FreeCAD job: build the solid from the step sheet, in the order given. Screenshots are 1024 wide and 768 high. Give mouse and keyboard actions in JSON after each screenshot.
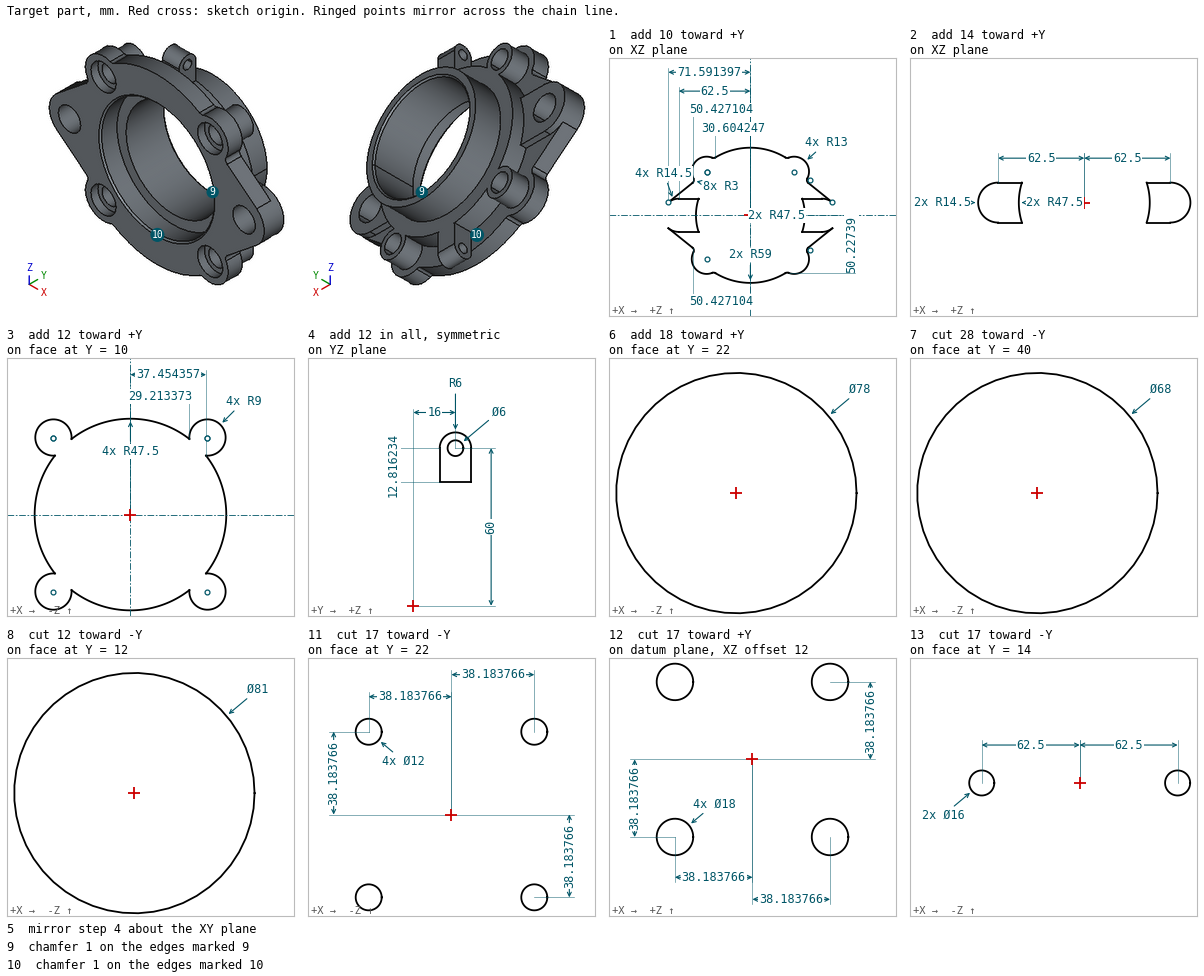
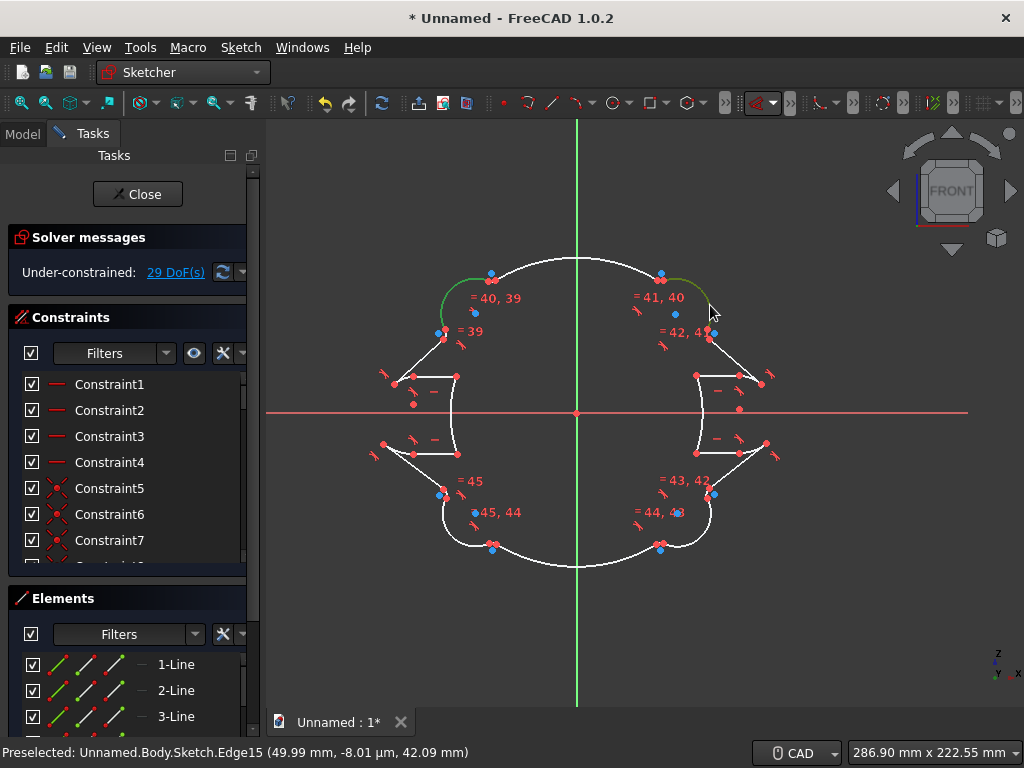
{"action": "left_click", "coordinate": [688, 545]}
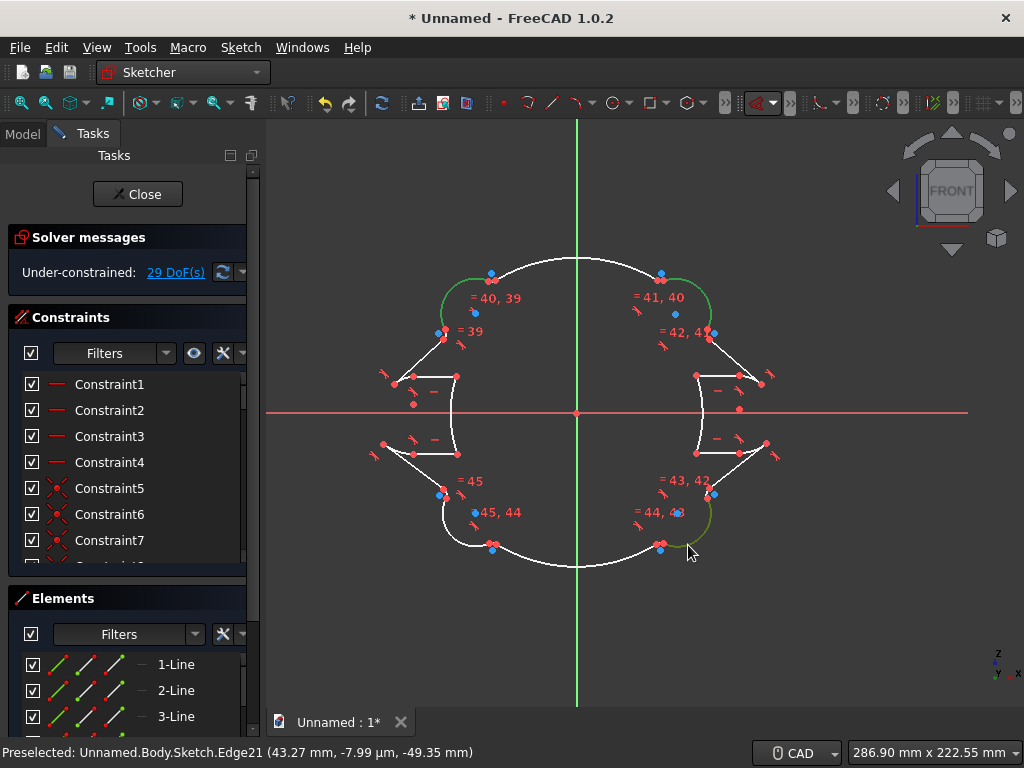
{"action": "left_click", "coordinate": [444, 522]}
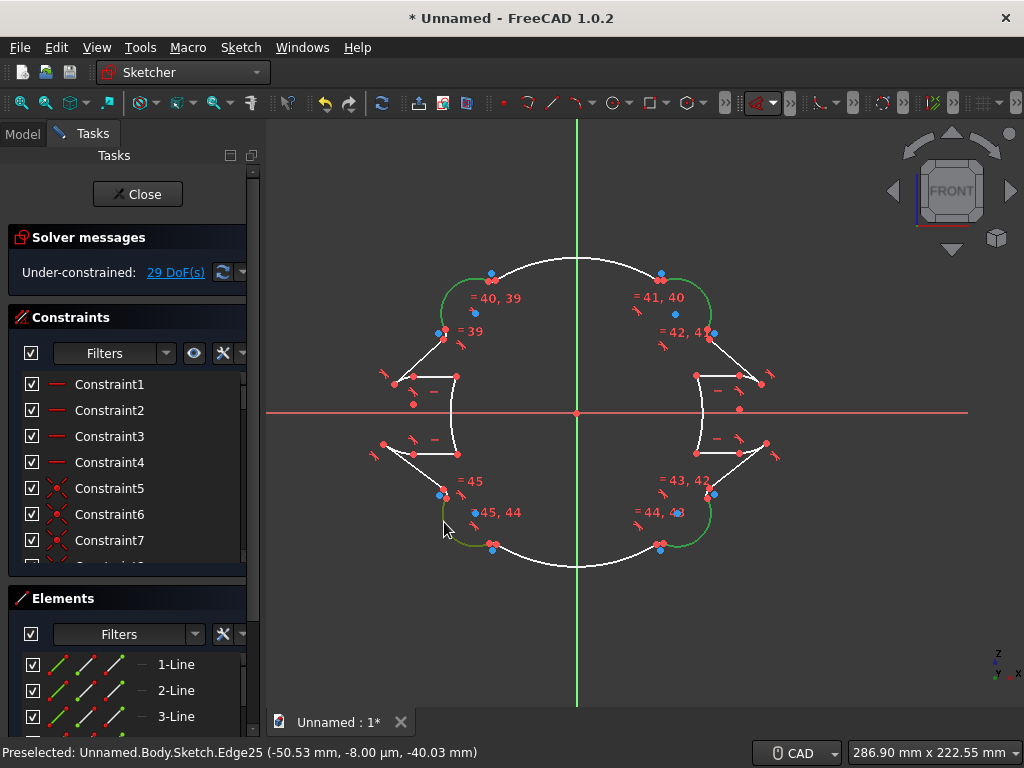
{"action": "key", "text": "e"}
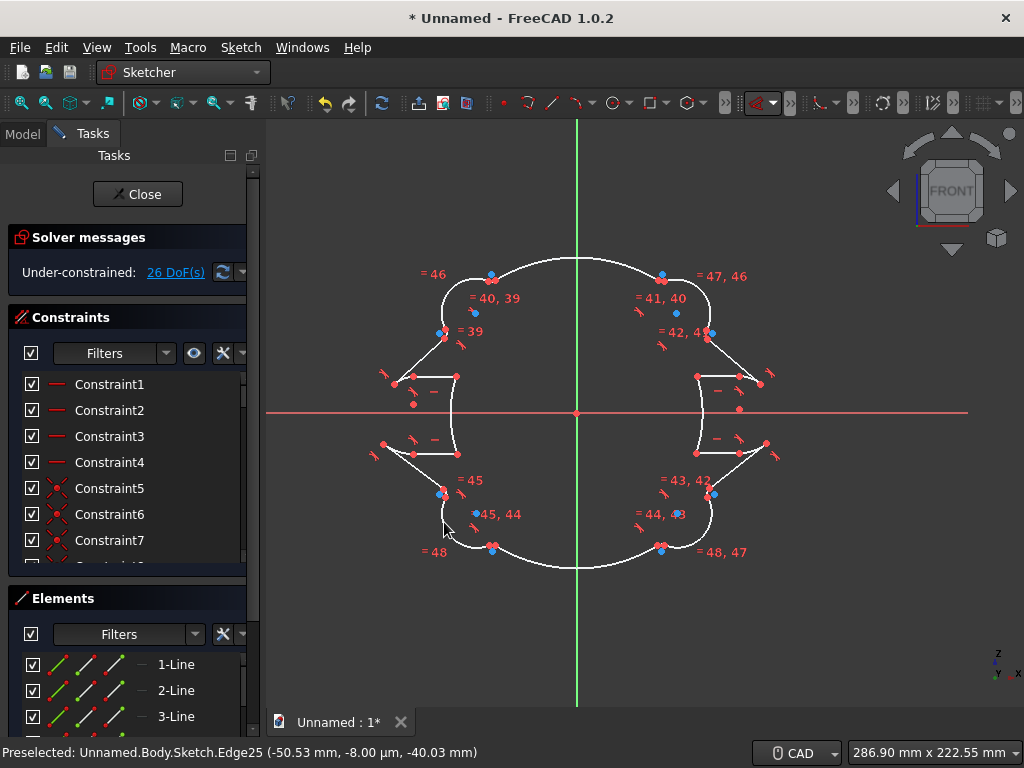
{"action": "scroll", "coordinate": [409, 377], "scroll_direction": "up", "scroll_amount": 7}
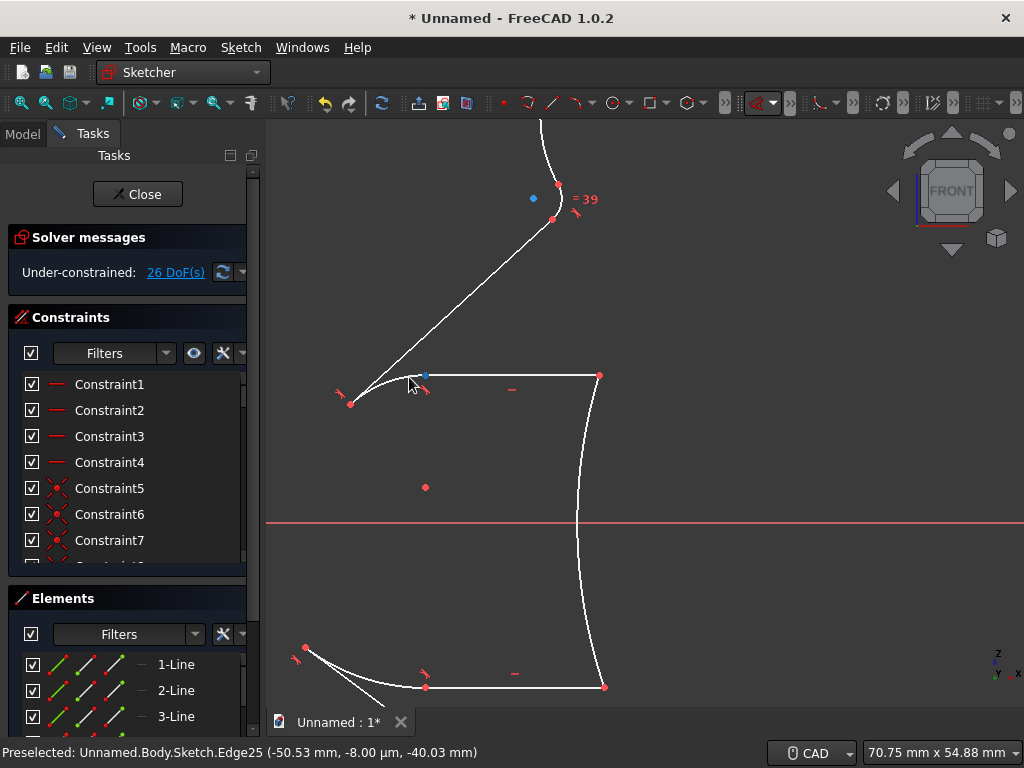
{"action": "left_click", "coordinate": [409, 376]}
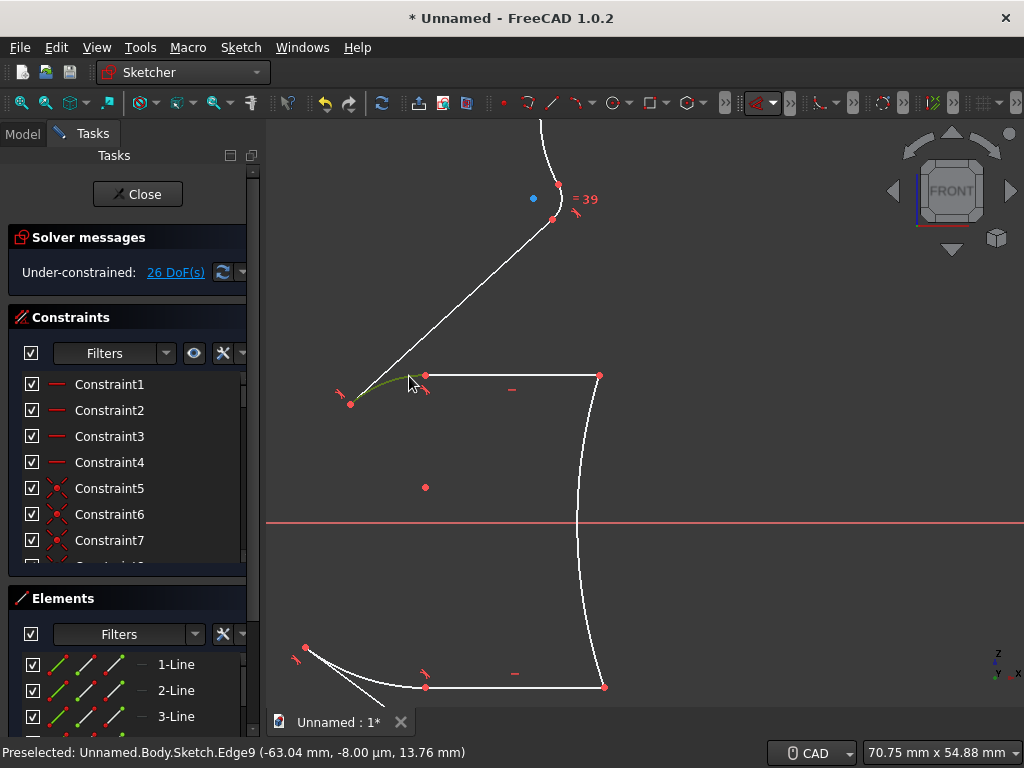
{"action": "scroll", "coordinate": [409, 377], "scroll_direction": "down", "scroll_amount": 7}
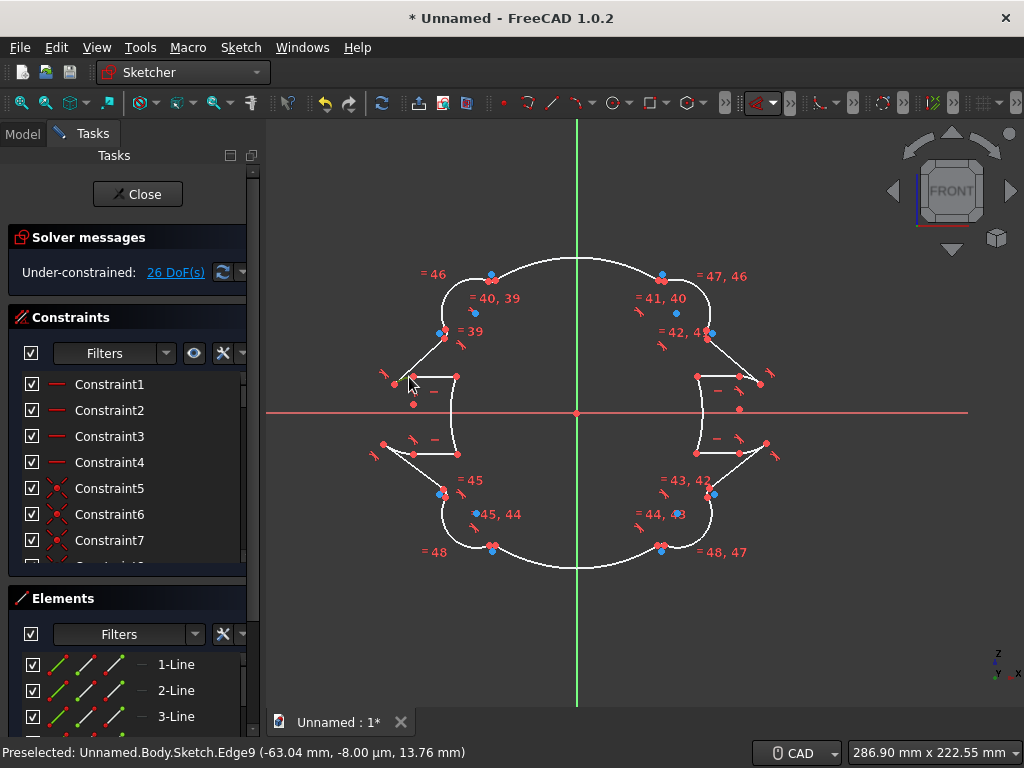
{"action": "scroll", "coordinate": [746, 377], "scroll_direction": "up", "scroll_amount": 7}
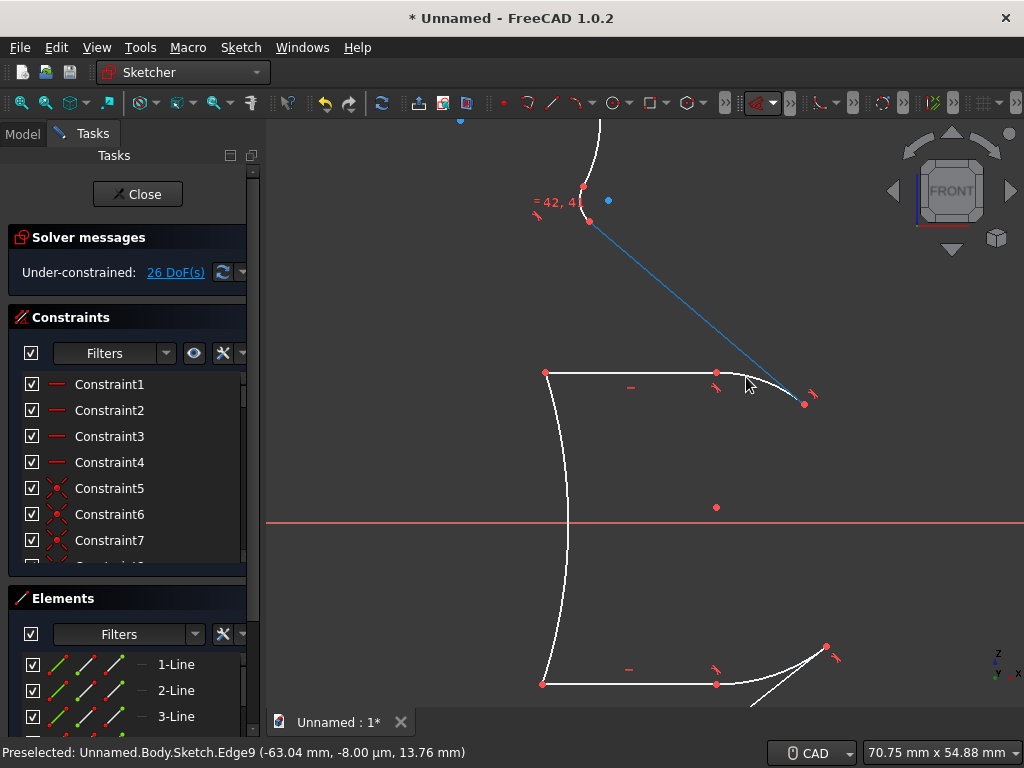
{"action": "left_click", "coordinate": [745, 376]}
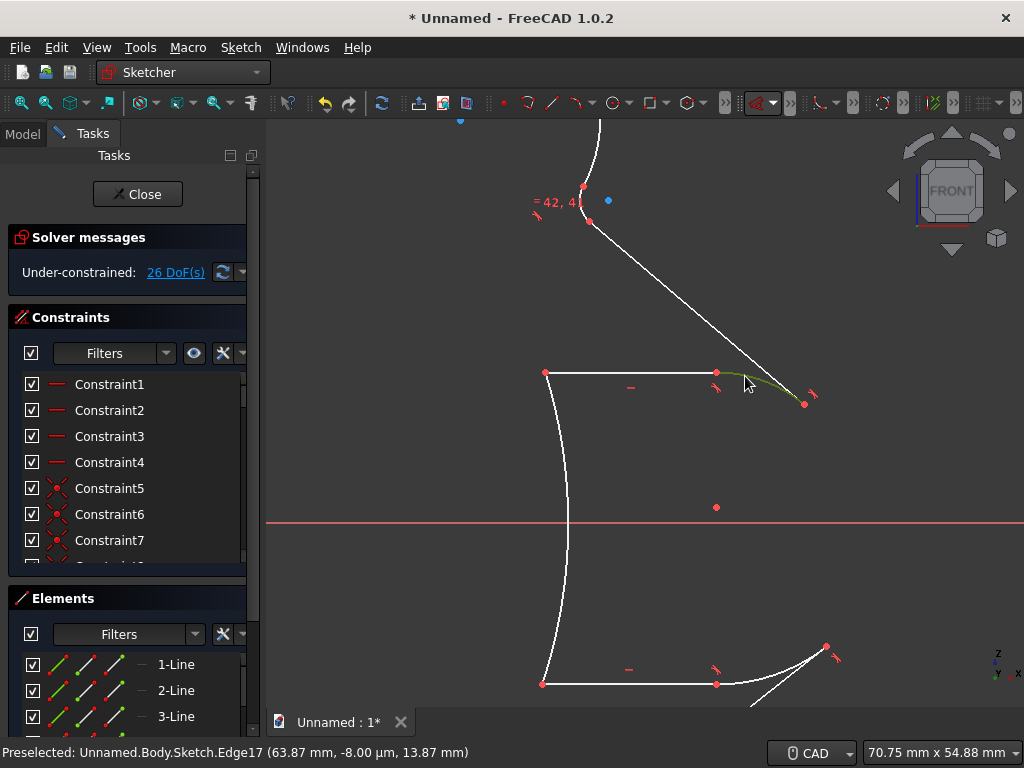
{"action": "scroll", "coordinate": [775, 675], "scroll_direction": "up", "scroll_amount": 2}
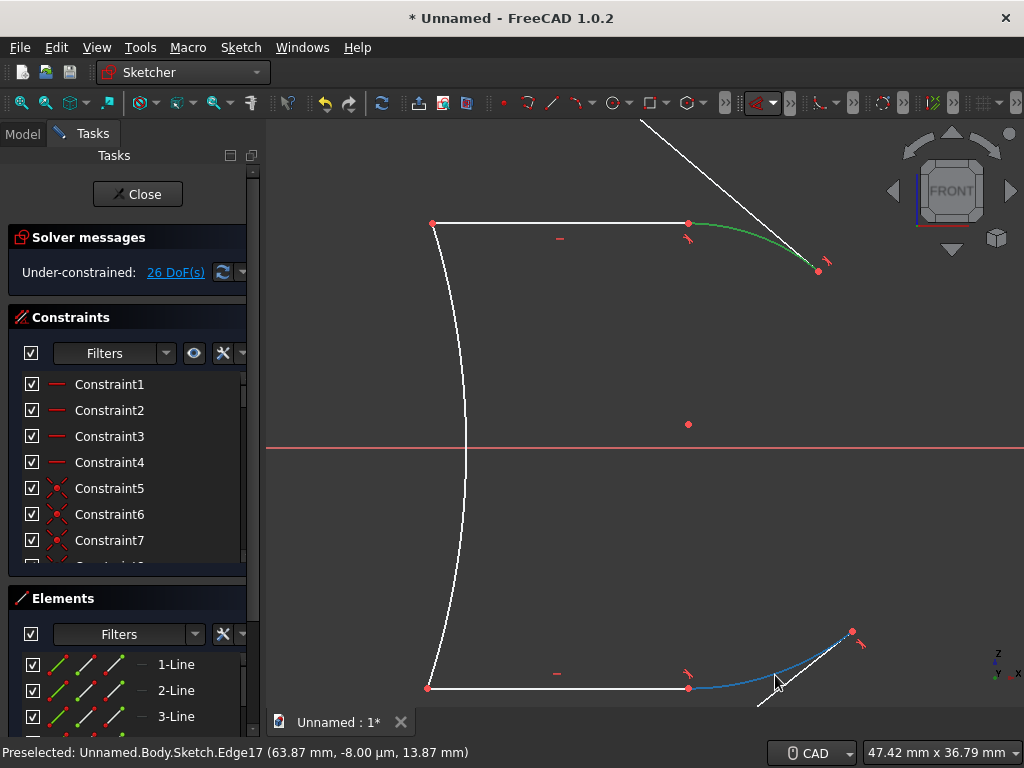
{"action": "left_click", "coordinate": [775, 674]}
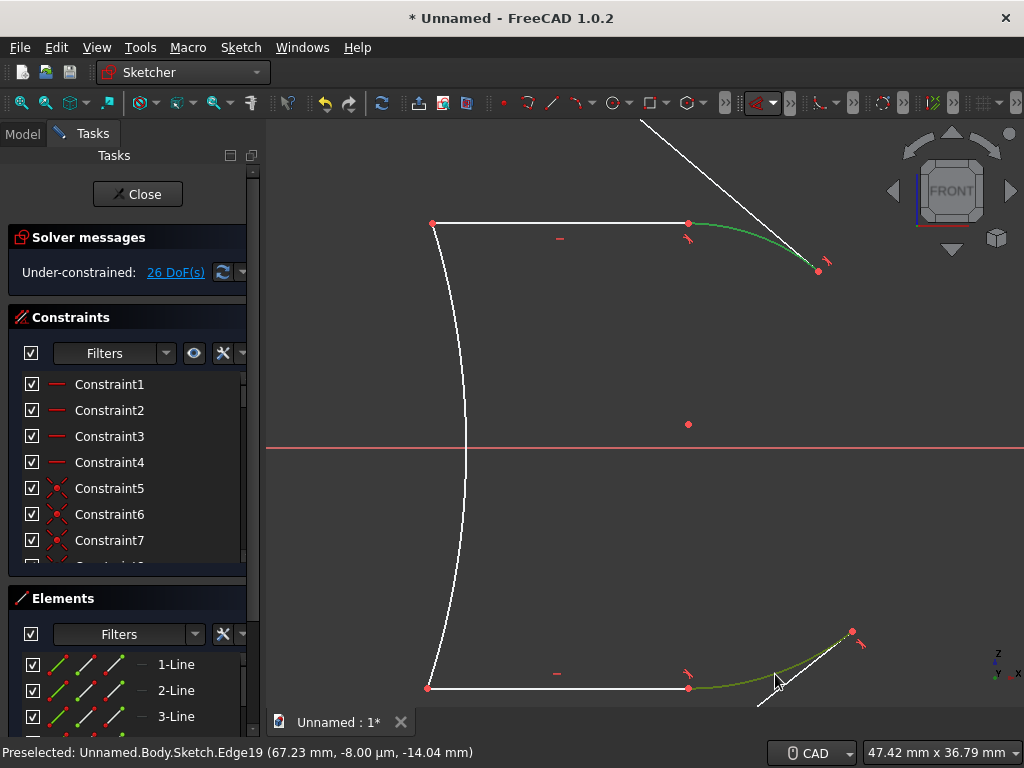
{"action": "scroll", "coordinate": [749, 406], "scroll_direction": "down", "scroll_amount": 9}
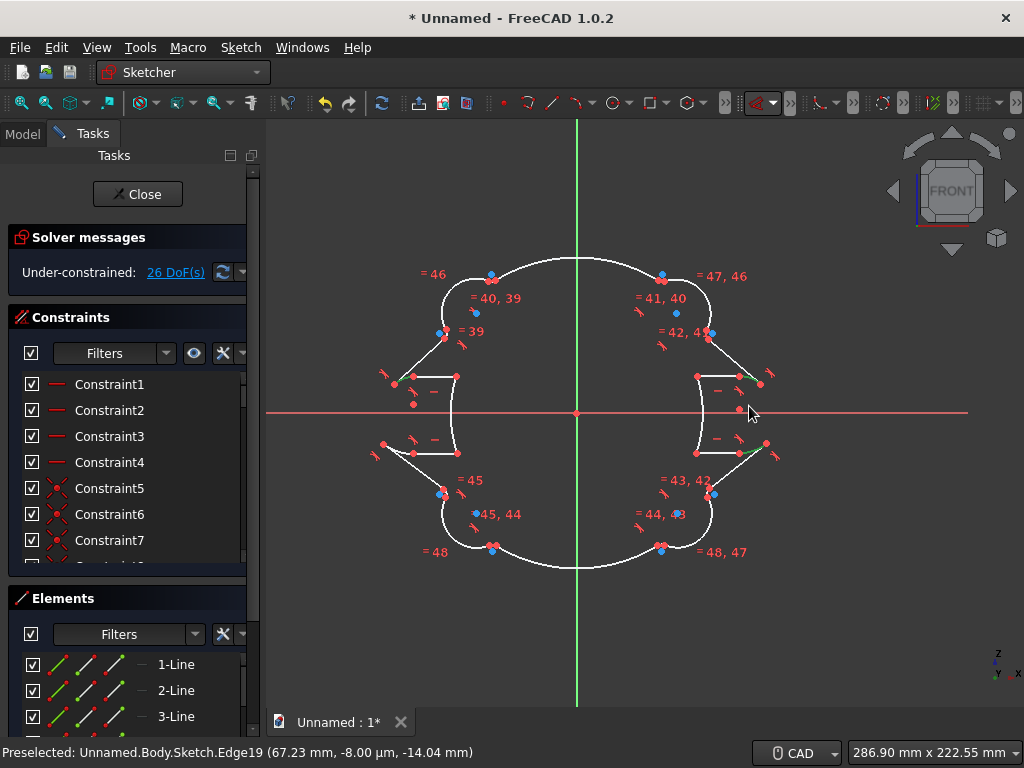
{"action": "scroll", "coordinate": [404, 453], "scroll_direction": "up", "scroll_amount": 6}